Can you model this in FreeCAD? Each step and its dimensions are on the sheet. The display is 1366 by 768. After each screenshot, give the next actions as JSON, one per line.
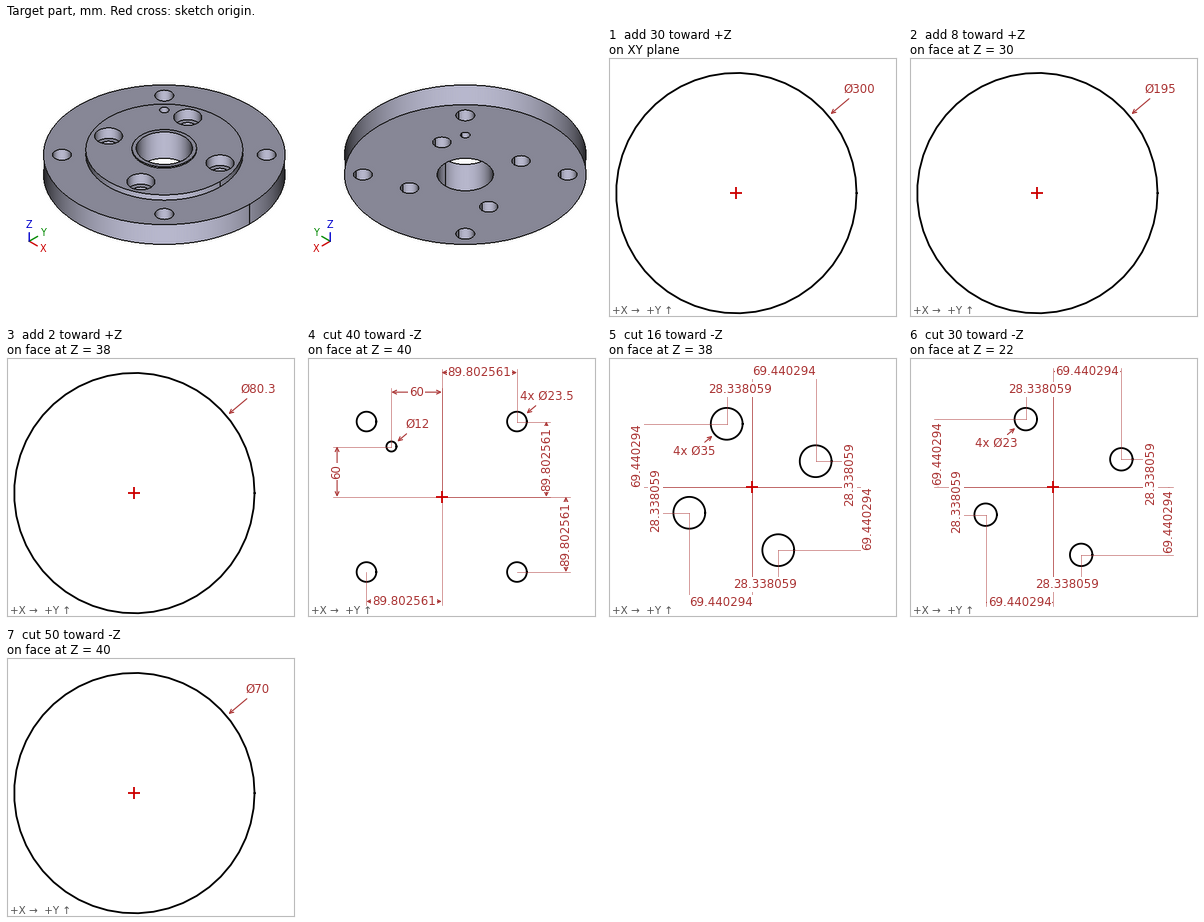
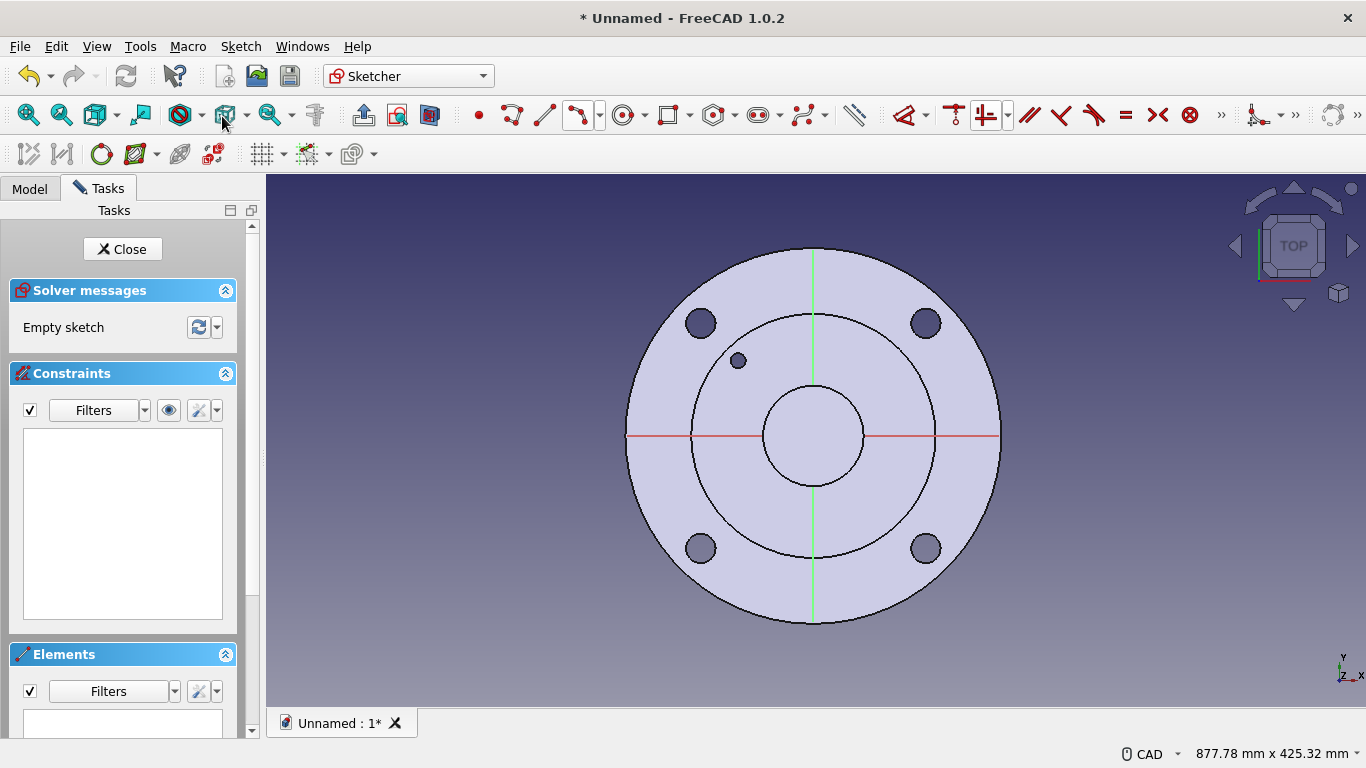
{"action": "scroll", "coordinate": [947, 427], "scroll_direction": "up", "scroll_amount": 2}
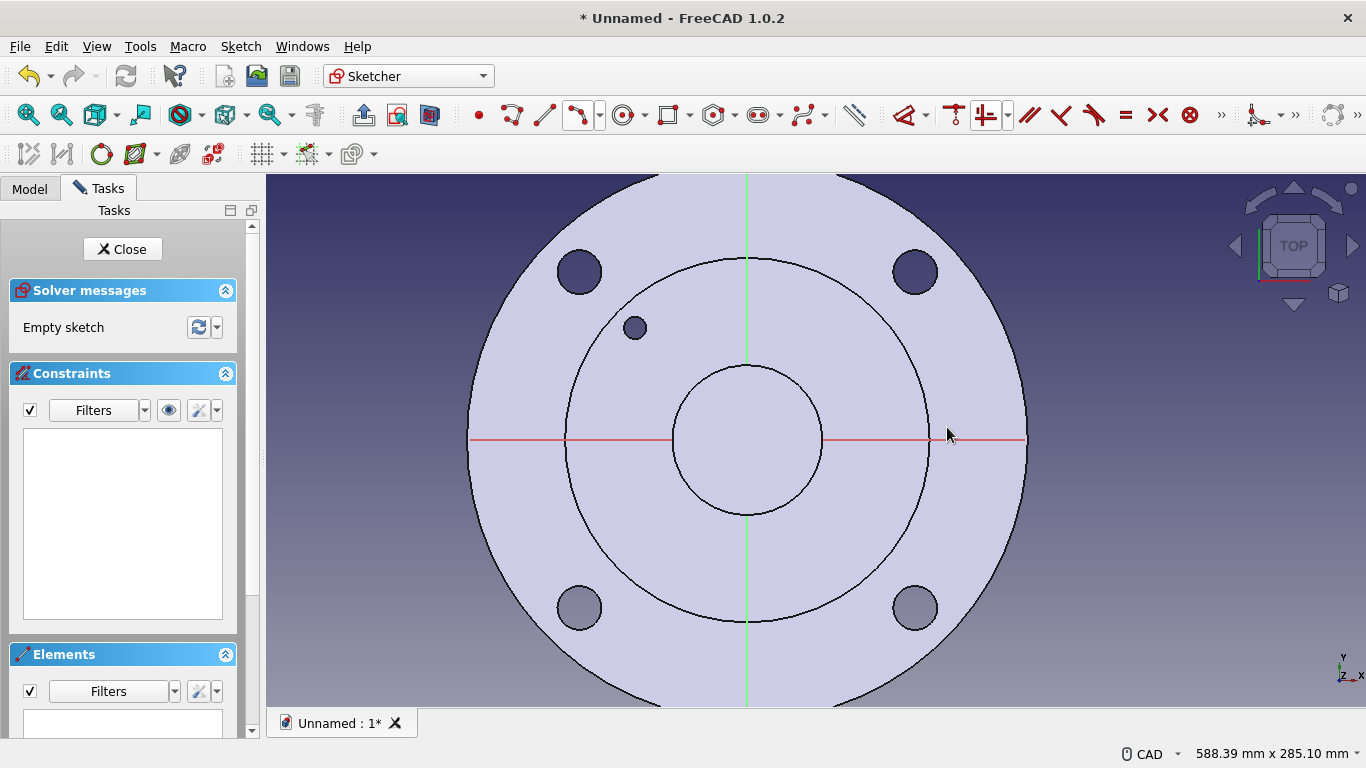
{"action": "left_click", "coordinate": [622, 116]}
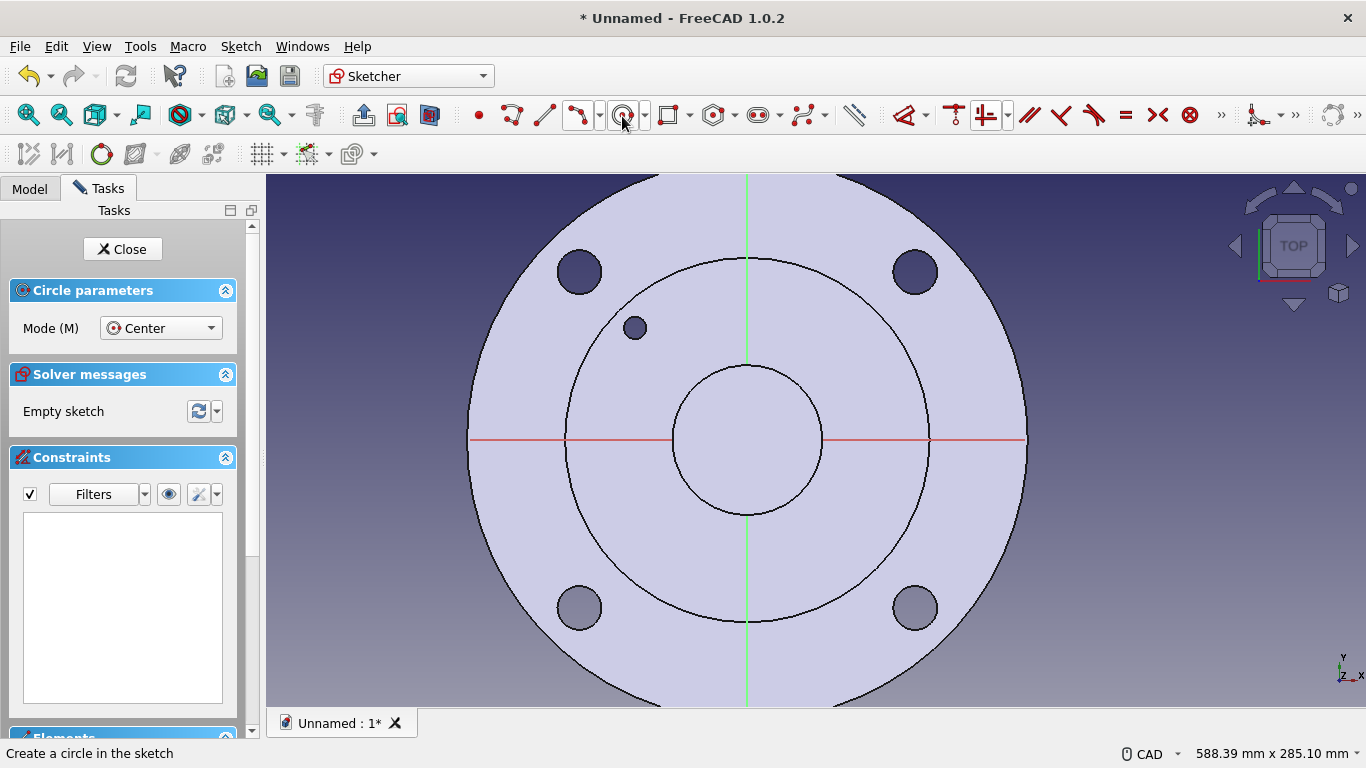
{"action": "left_click", "coordinate": [694, 310]}
{"action": "left_click", "coordinate": [717, 287]}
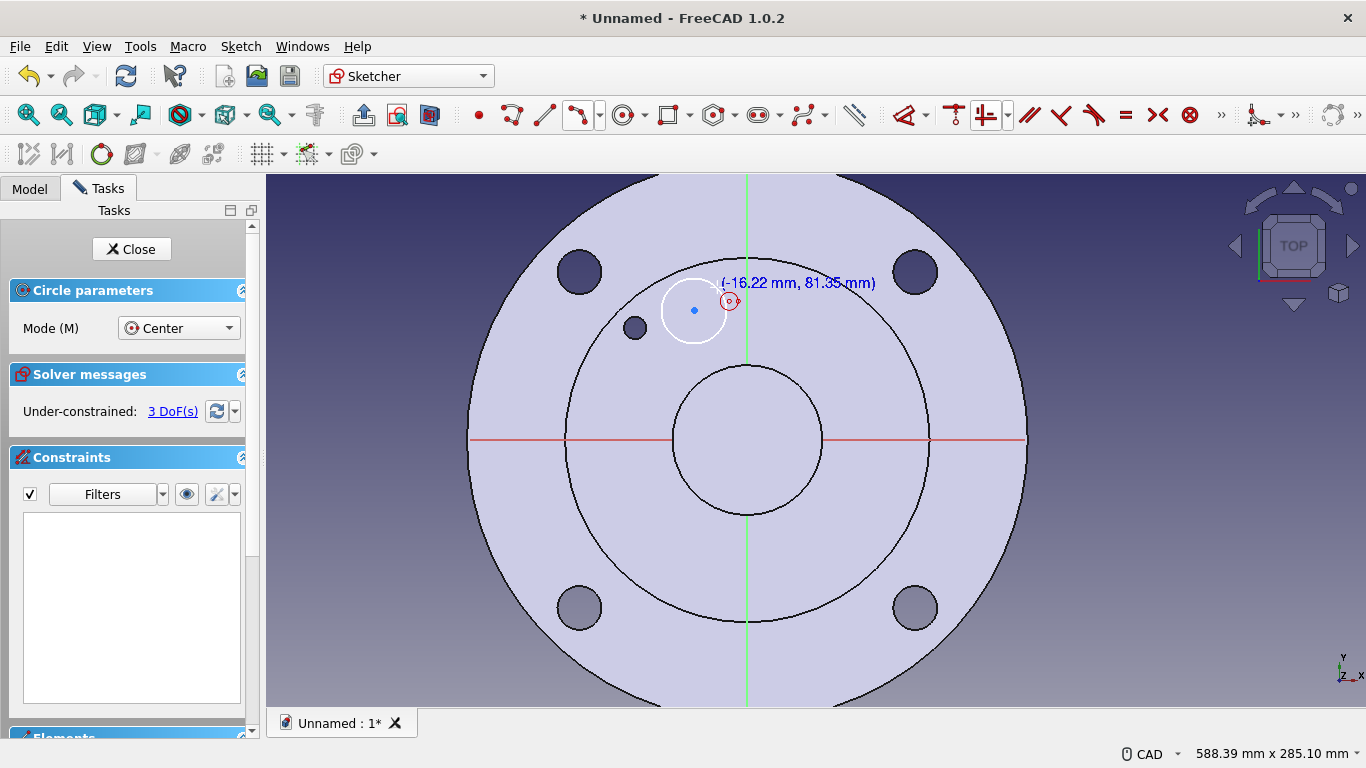
{"action": "left_click", "coordinate": [877, 387]}
{"action": "left_click", "coordinate": [900, 364]}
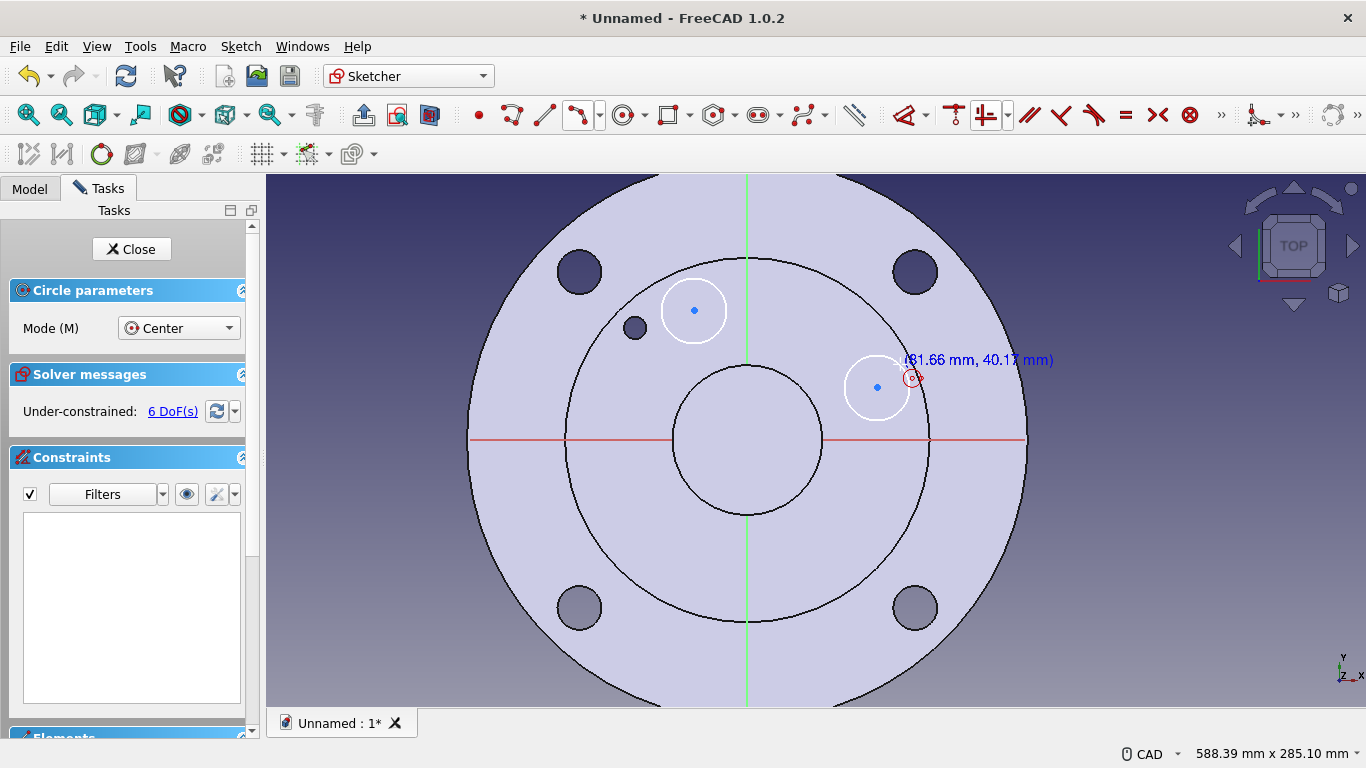
{"action": "left_click", "coordinate": [800, 570]}
{"action": "left_click", "coordinate": [823, 547]}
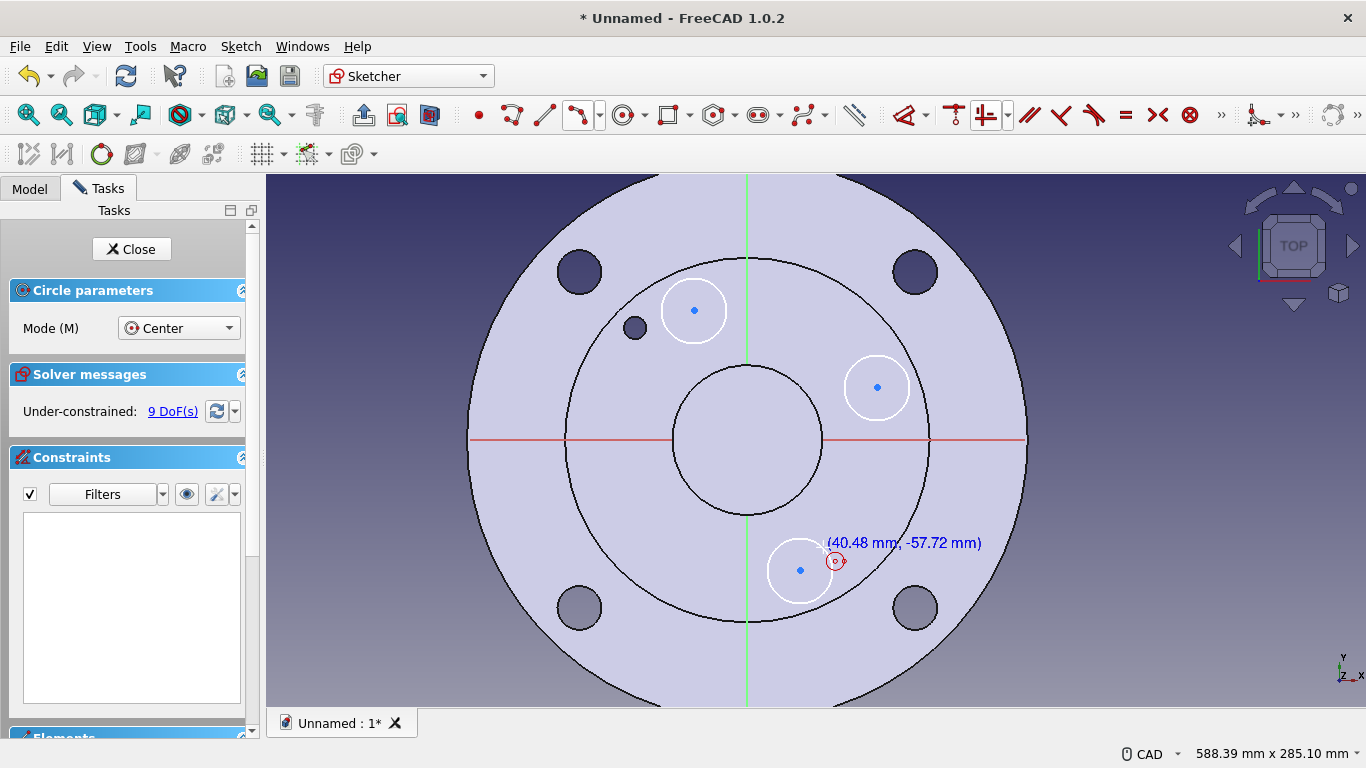
{"action": "left_click", "coordinate": [618, 493]}
{"action": "left_click", "coordinate": [641, 470]}
{"action": "key", "text": "Escape"}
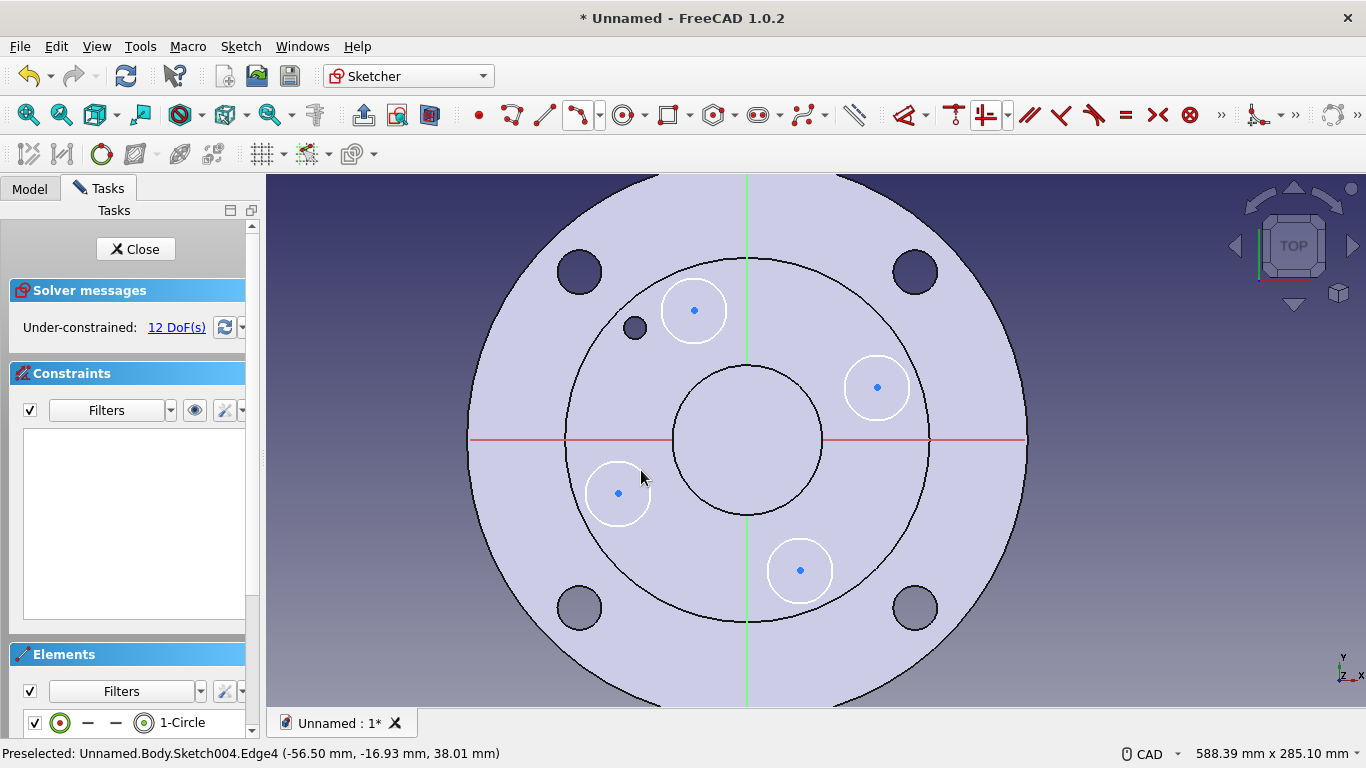
{"action": "left_click", "coordinate": [717, 288]}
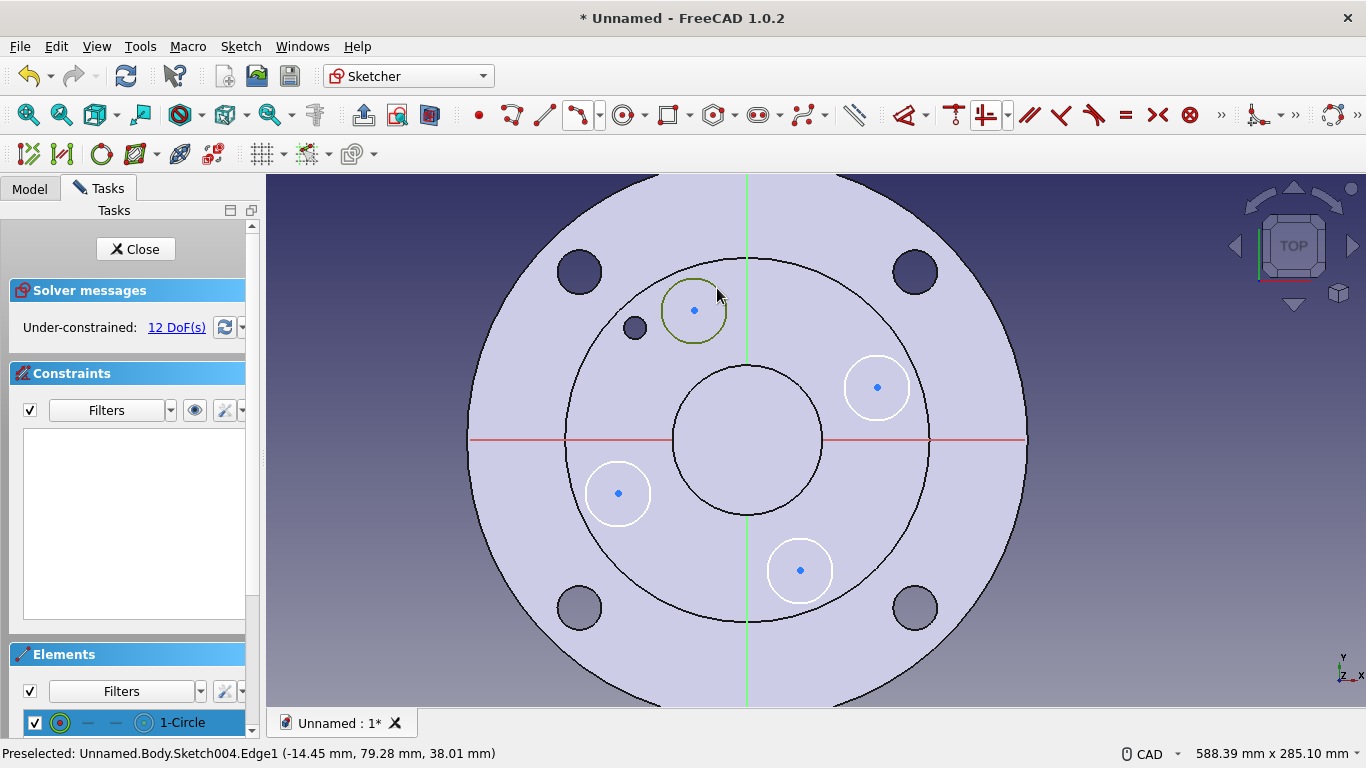
{"action": "left_click", "coordinate": [900, 365]}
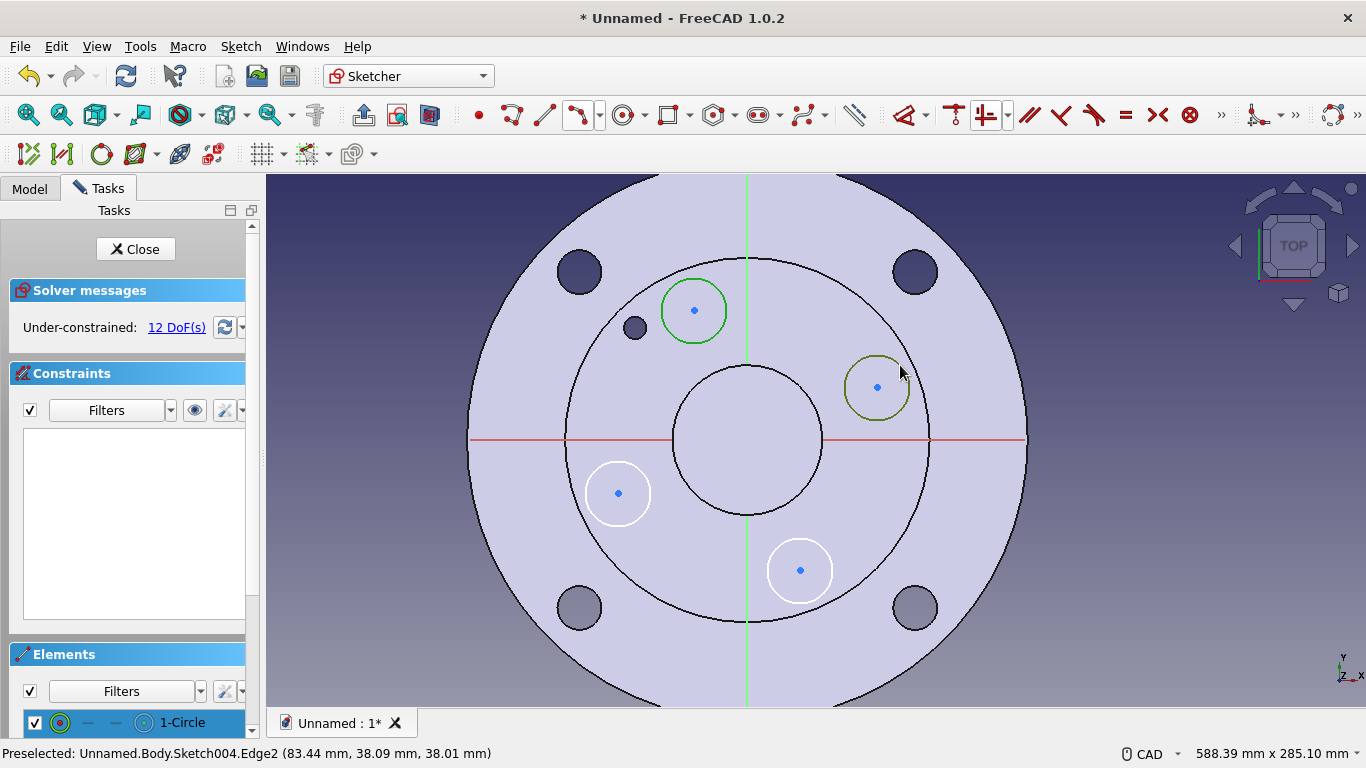
{"action": "left_click", "coordinate": [823, 548]}